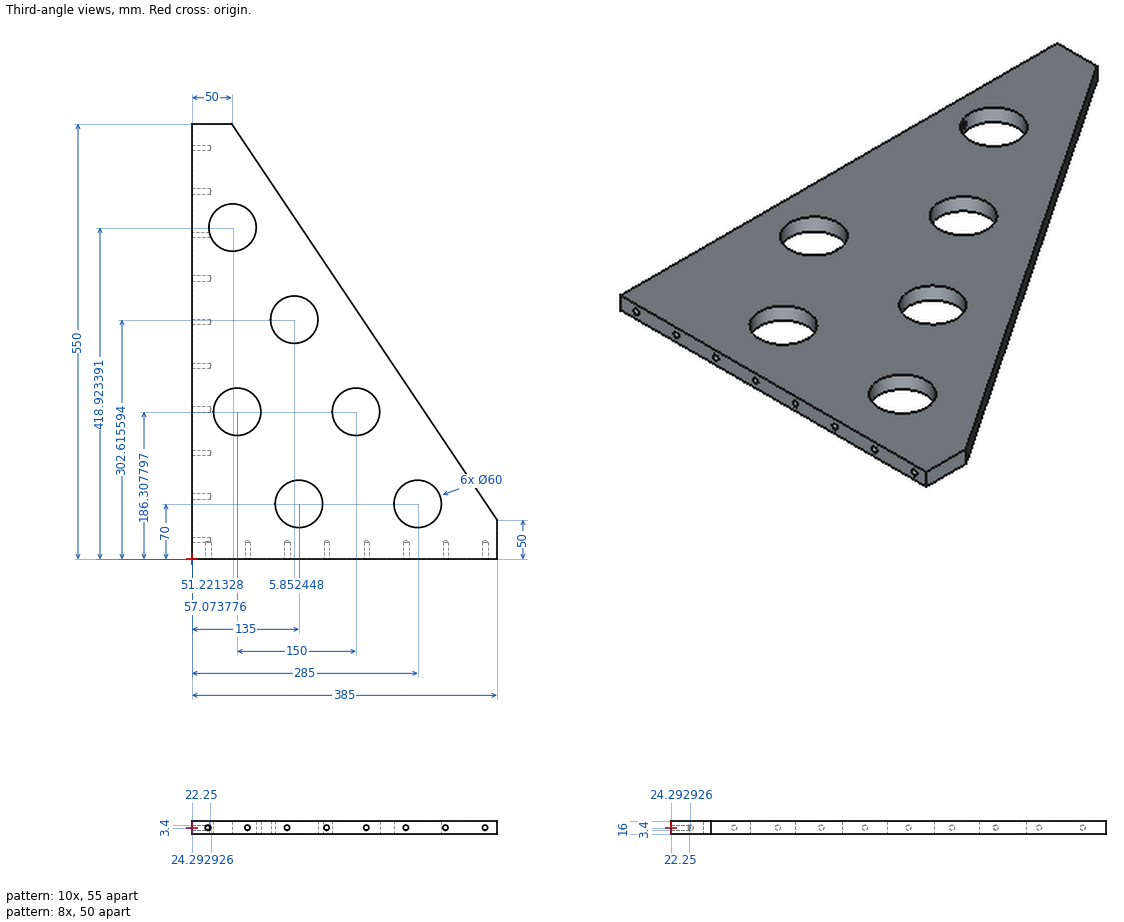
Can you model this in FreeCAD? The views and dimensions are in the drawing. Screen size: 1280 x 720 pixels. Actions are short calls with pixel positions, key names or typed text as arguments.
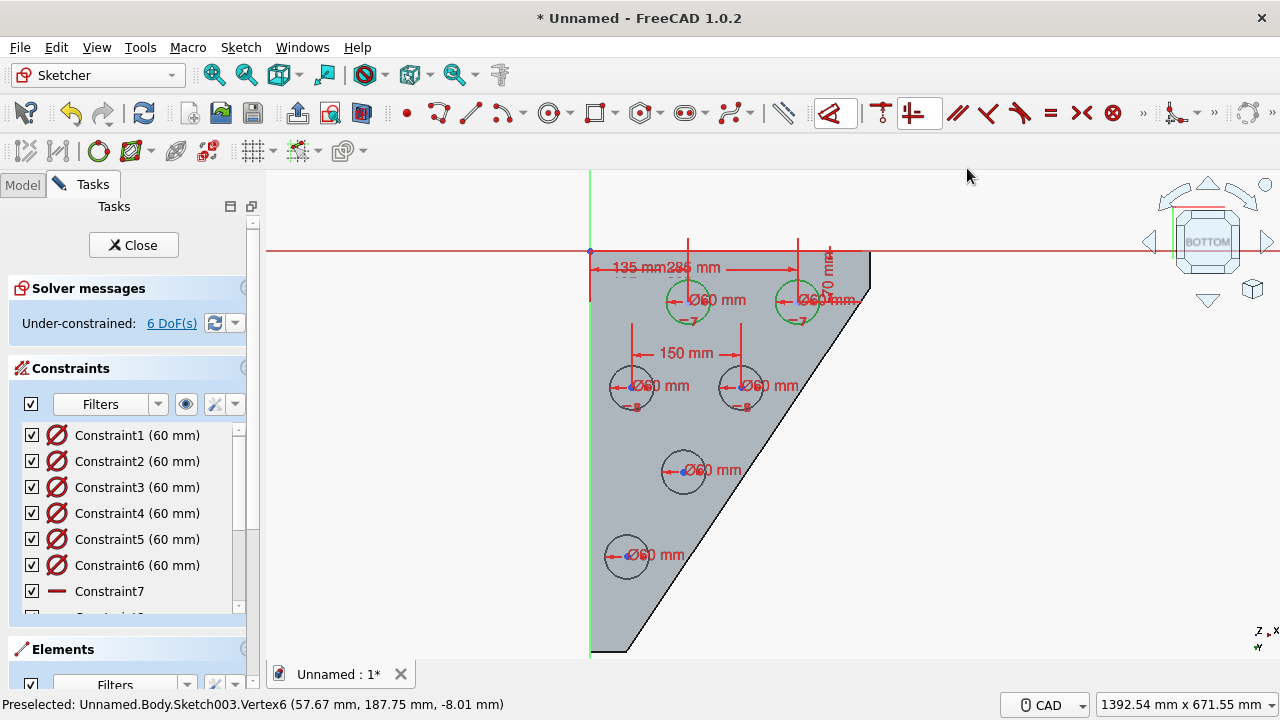
click(627, 557)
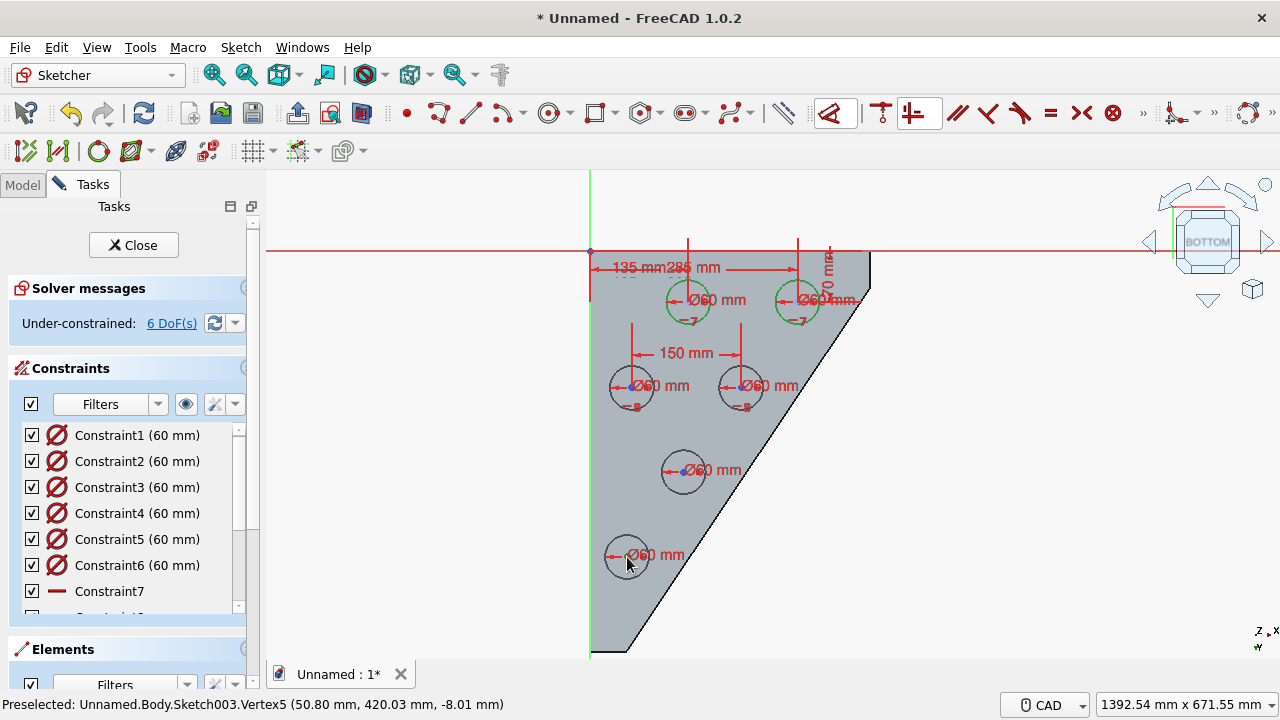
click(852, 114)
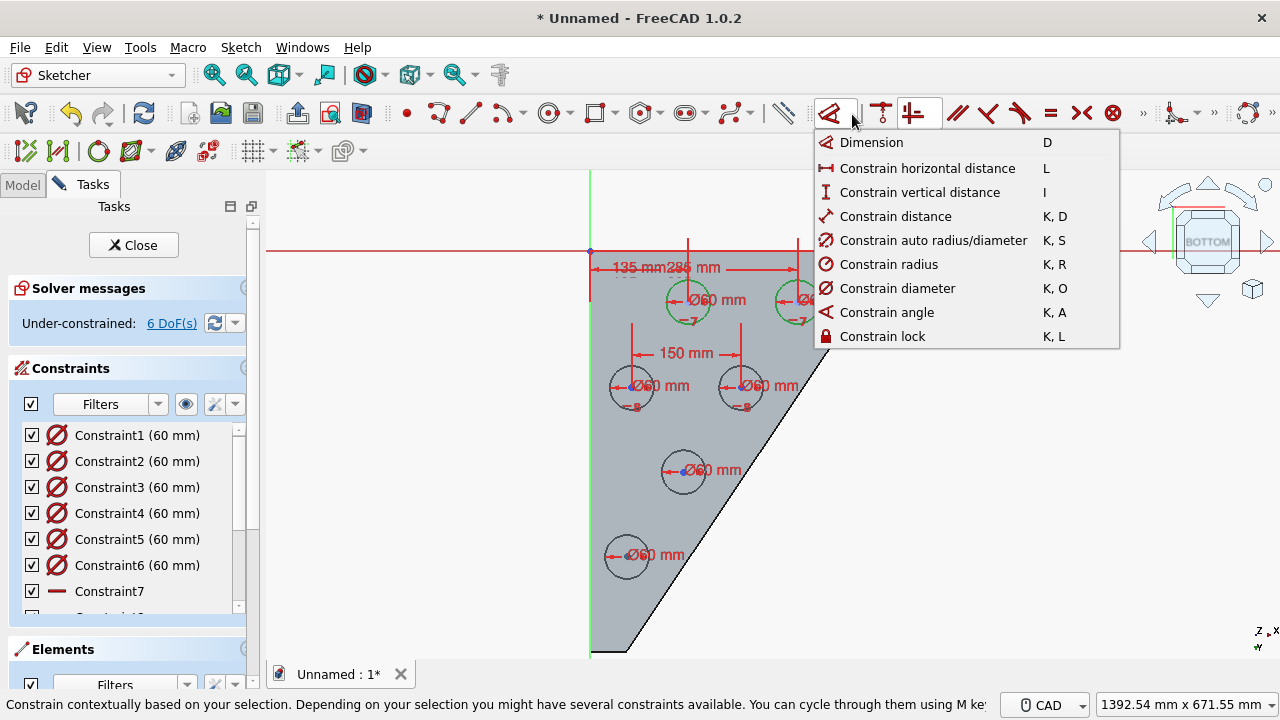
click(967, 168)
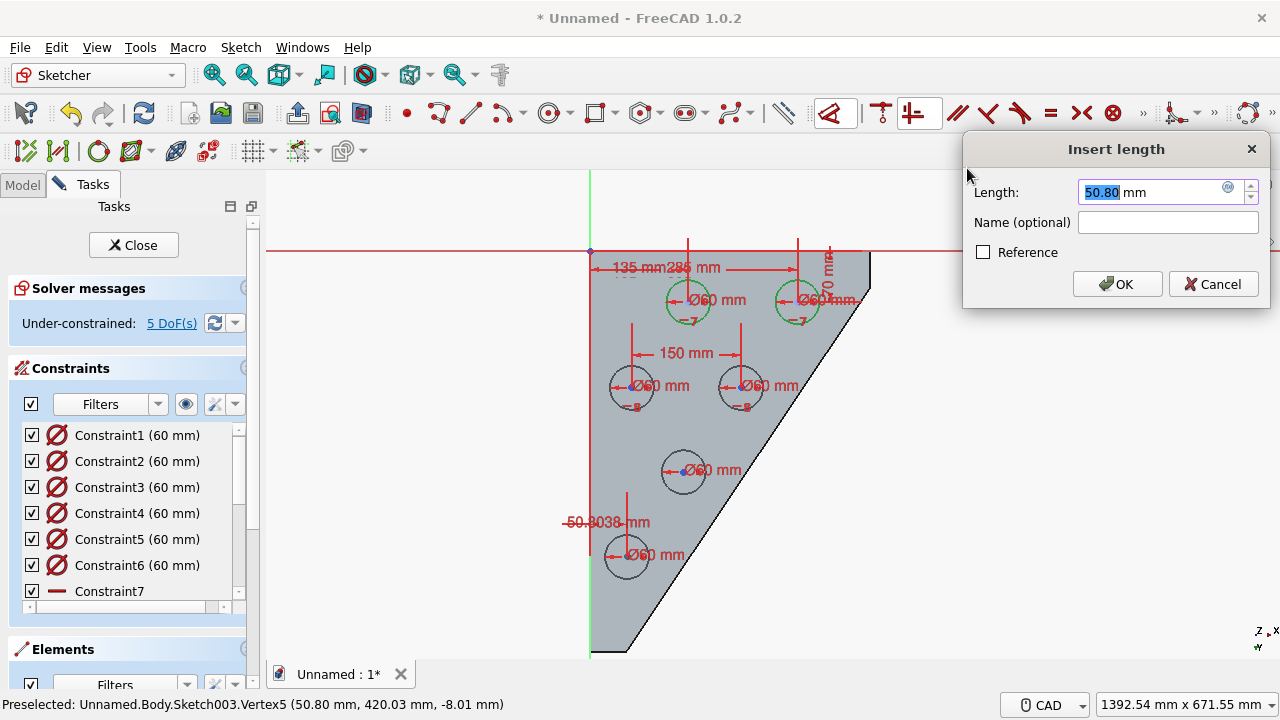
text(51.221328)
key(Return)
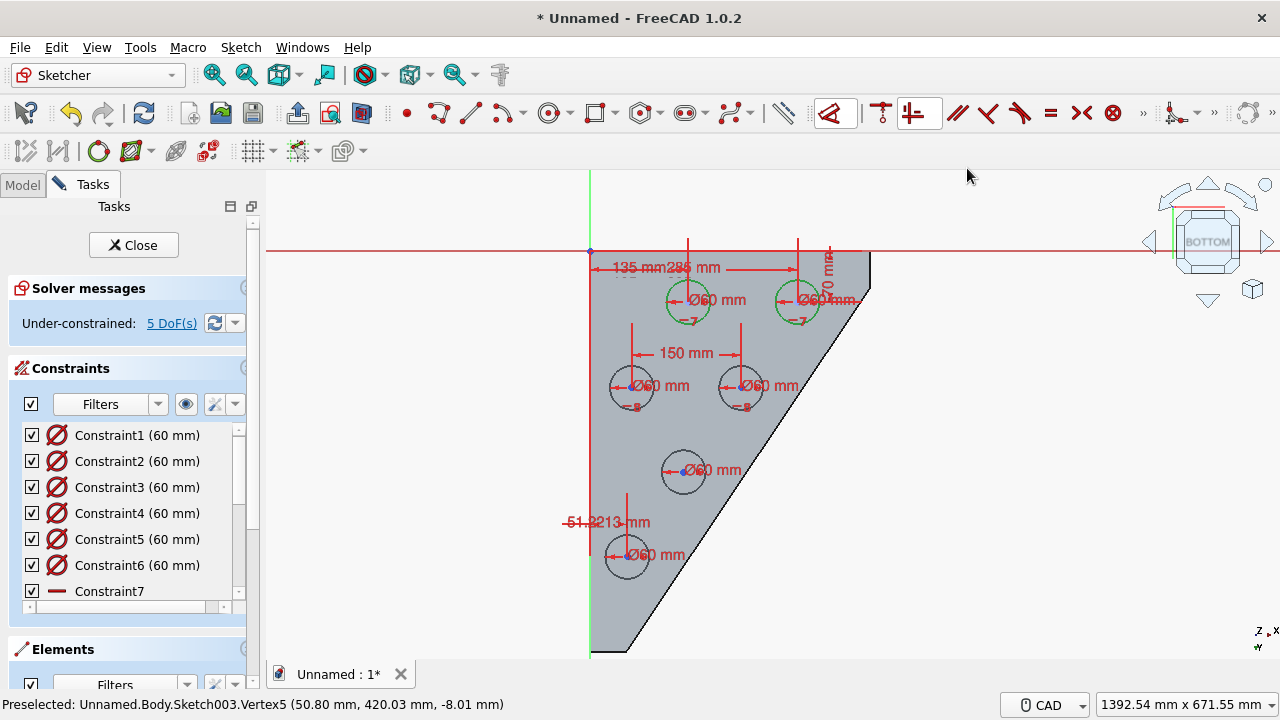
click(632, 388)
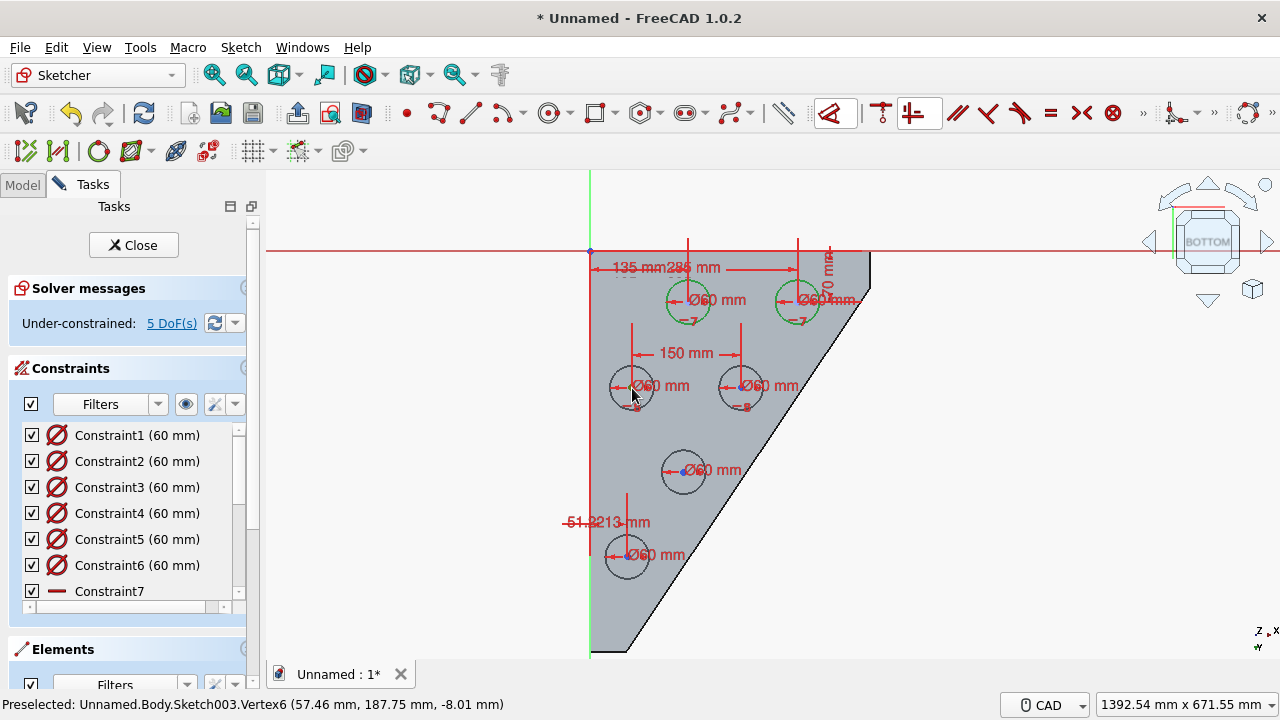
key(l)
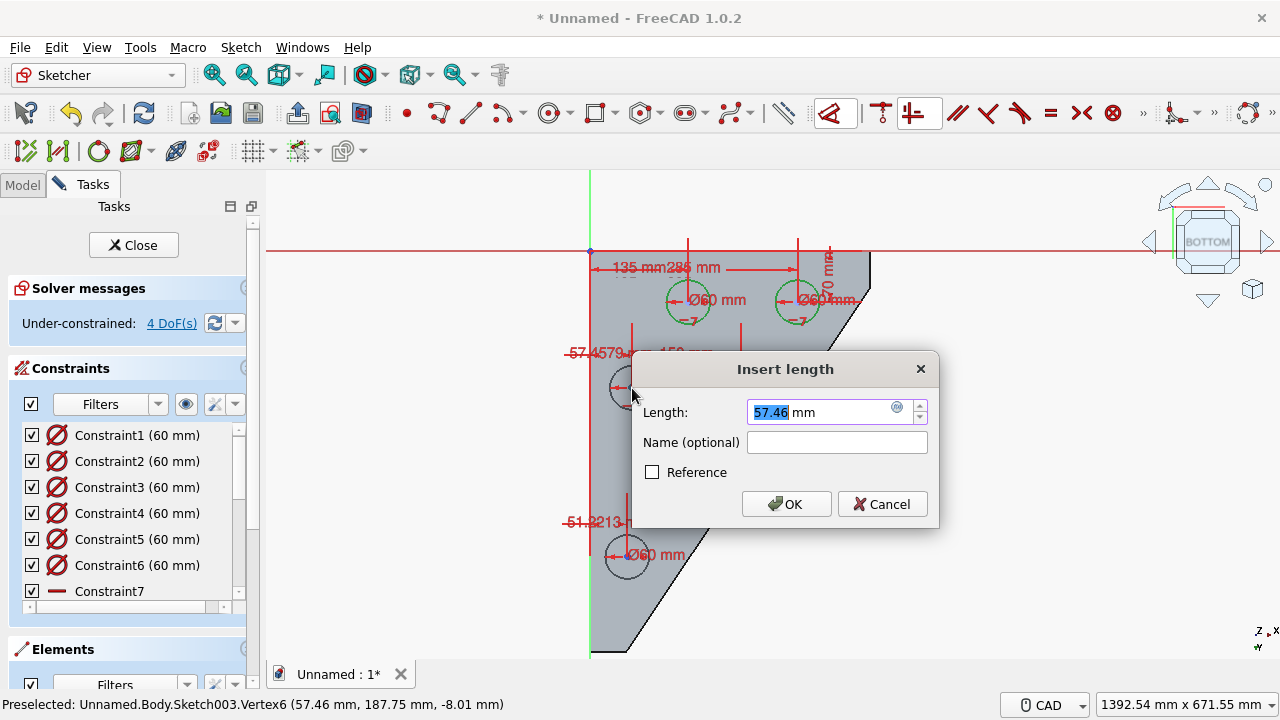
text(57.073776)
key(Return)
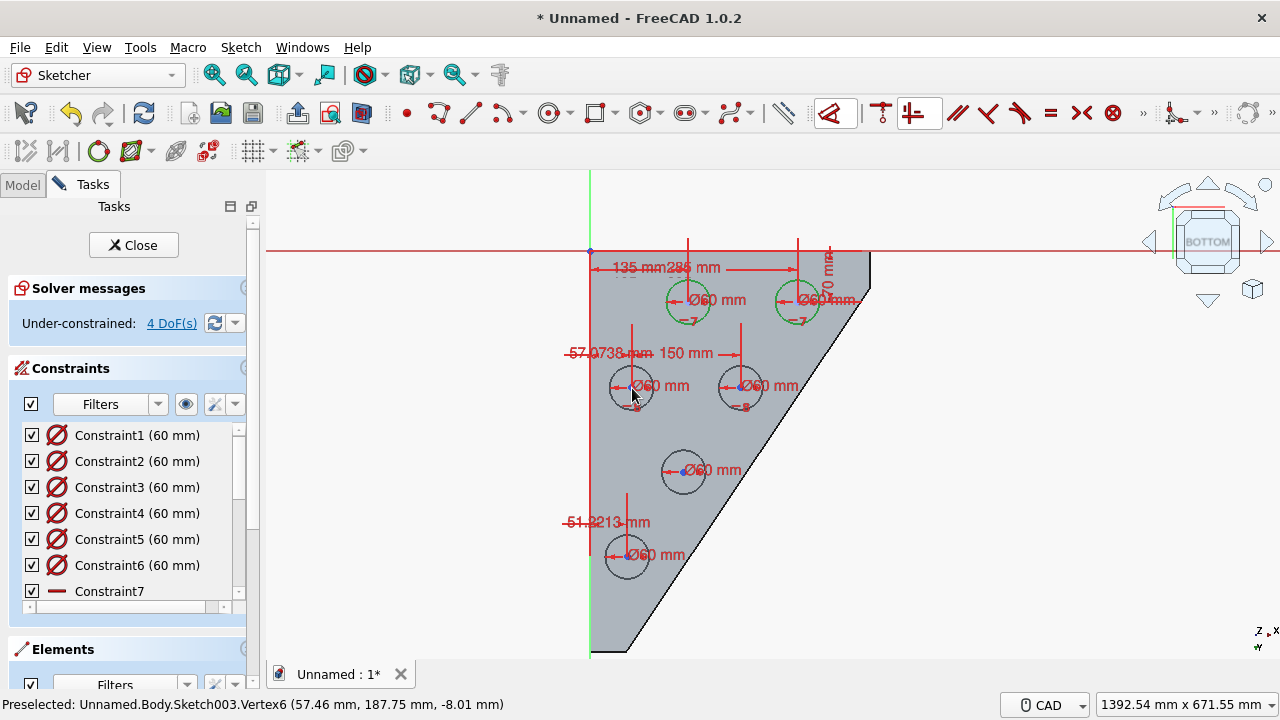
scroll(684, 472, up, 12)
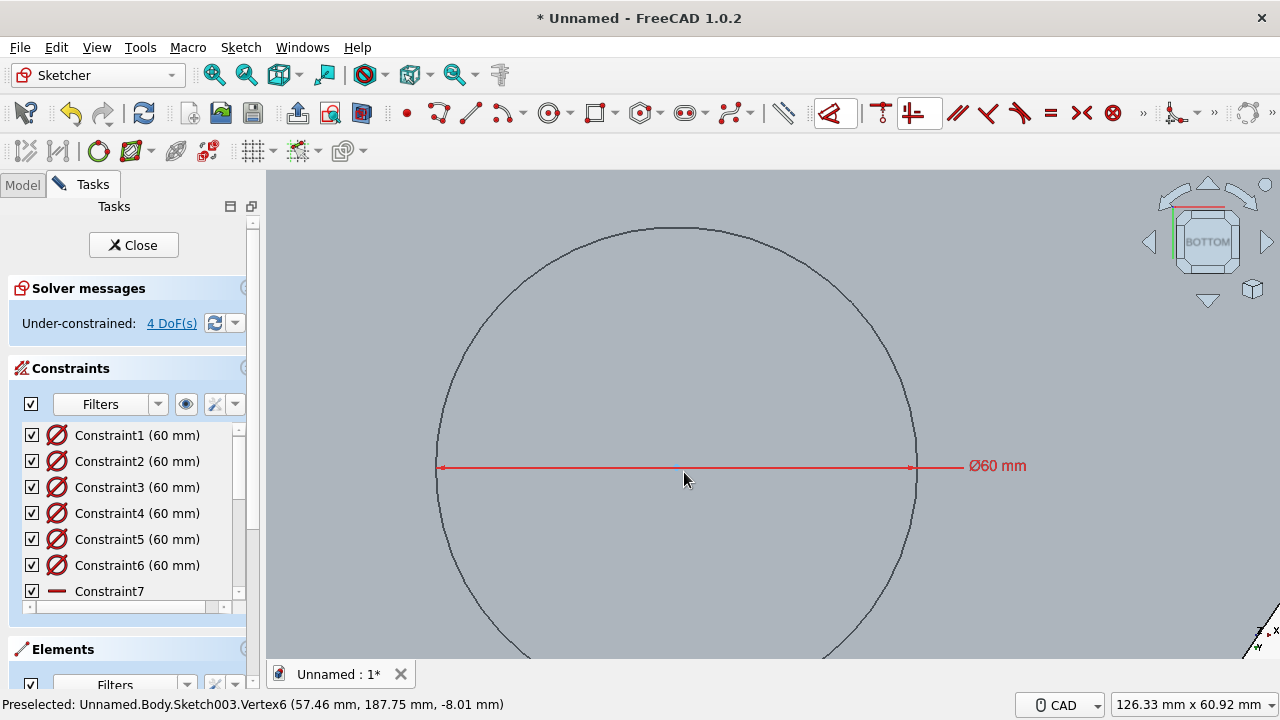
click(677, 468)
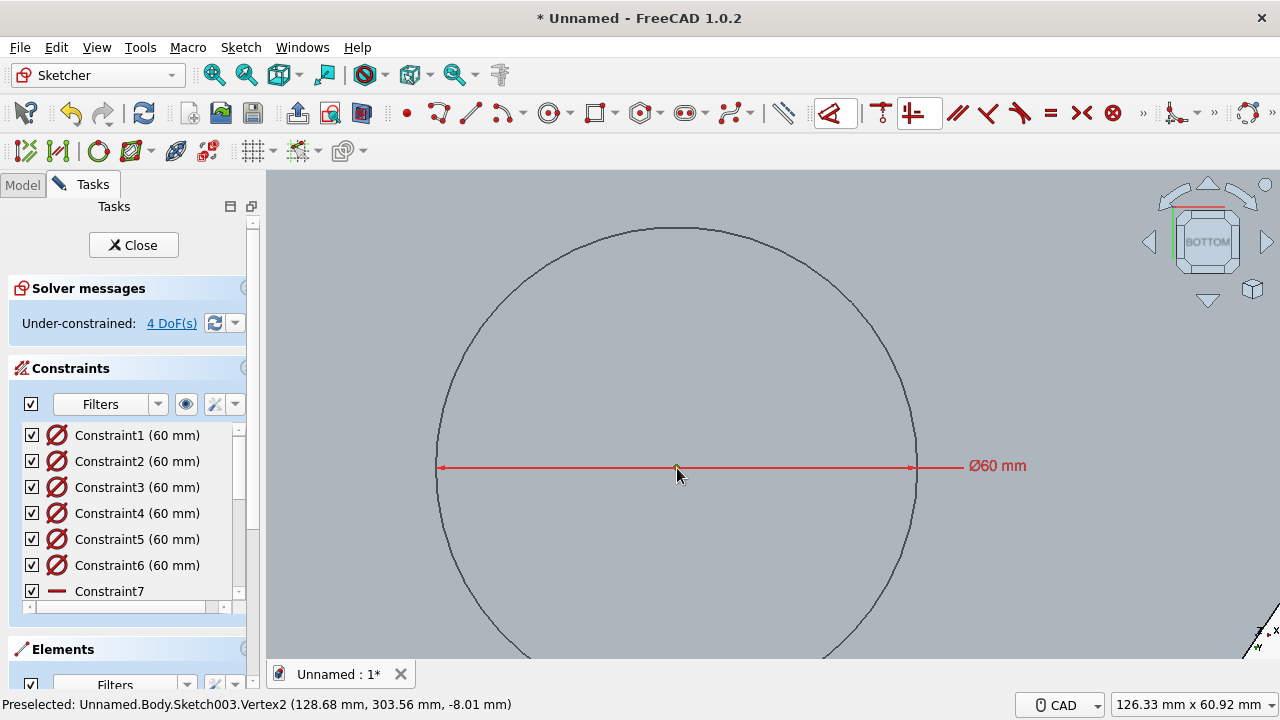
scroll(684, 473, down, 12)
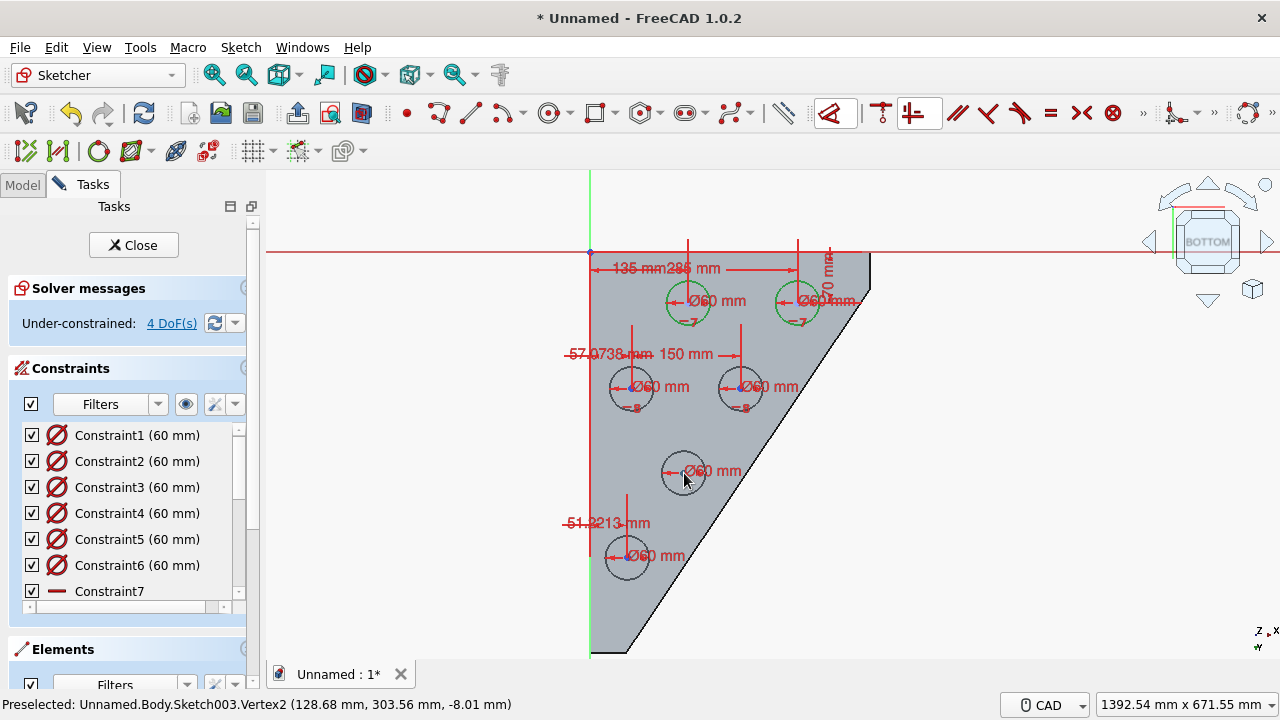
scroll(688, 303, up, 12)